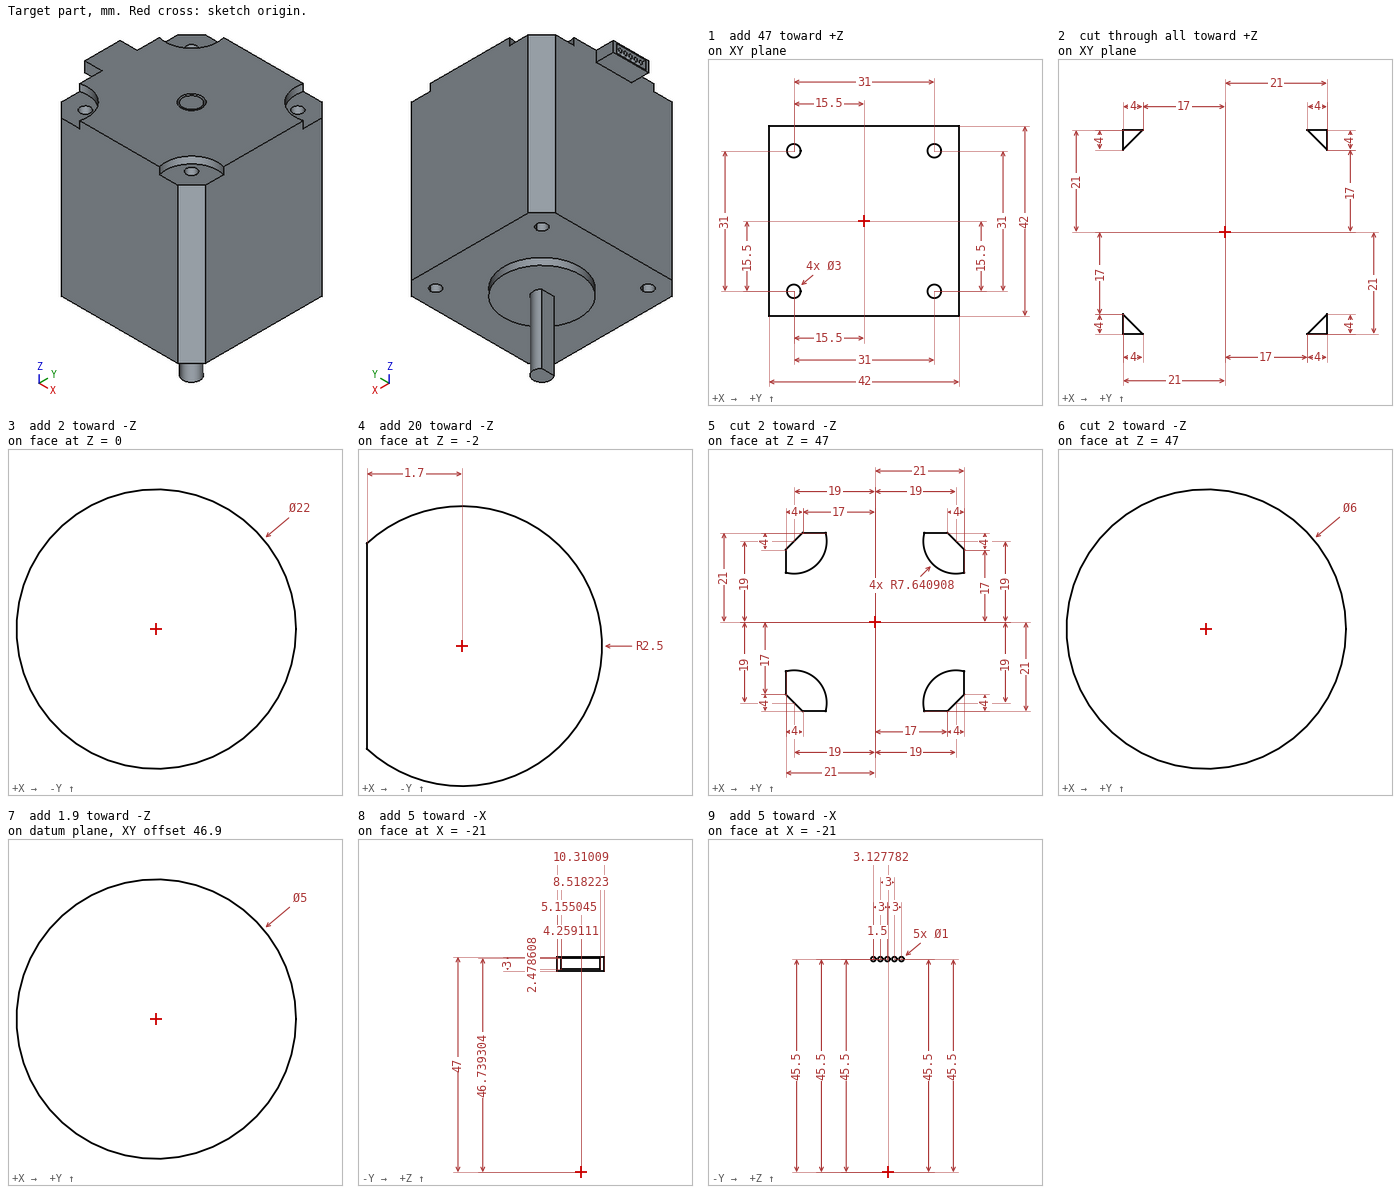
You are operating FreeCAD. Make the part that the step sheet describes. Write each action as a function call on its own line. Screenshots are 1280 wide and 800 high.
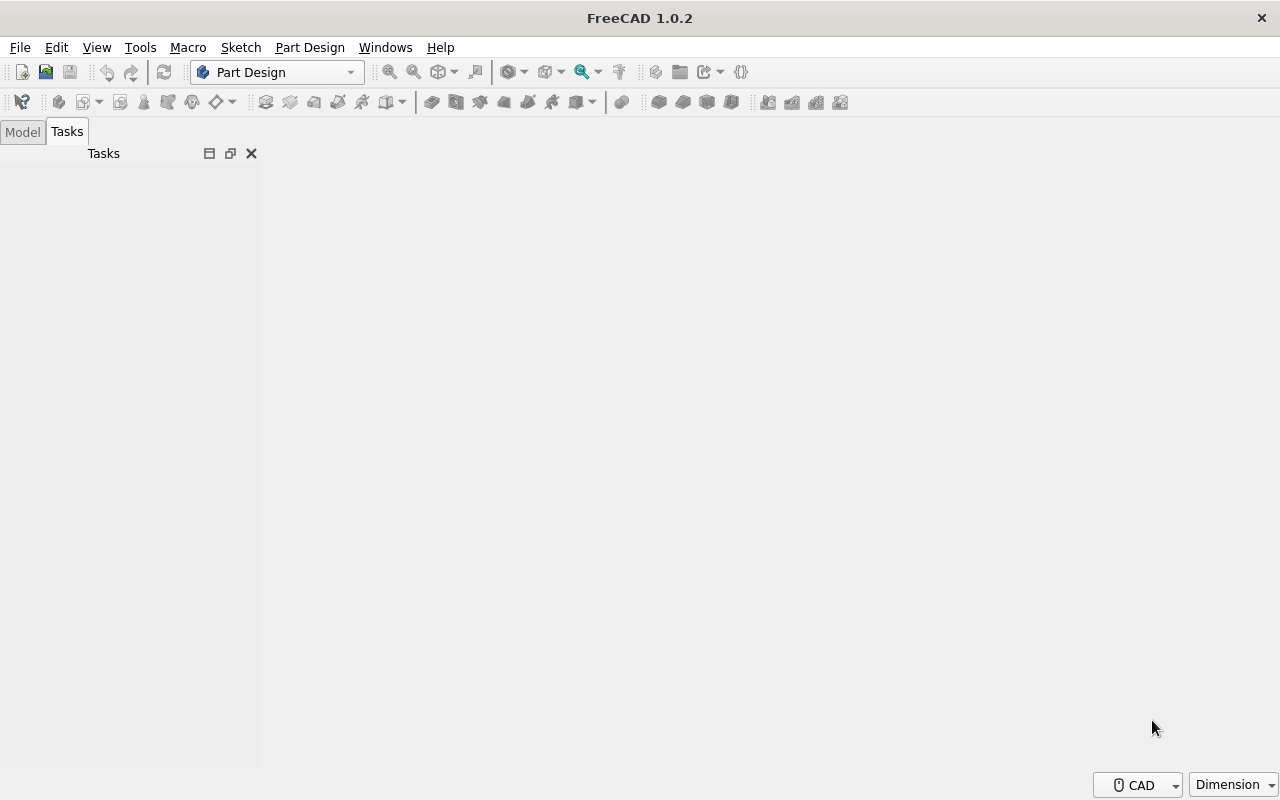
click(22, 72)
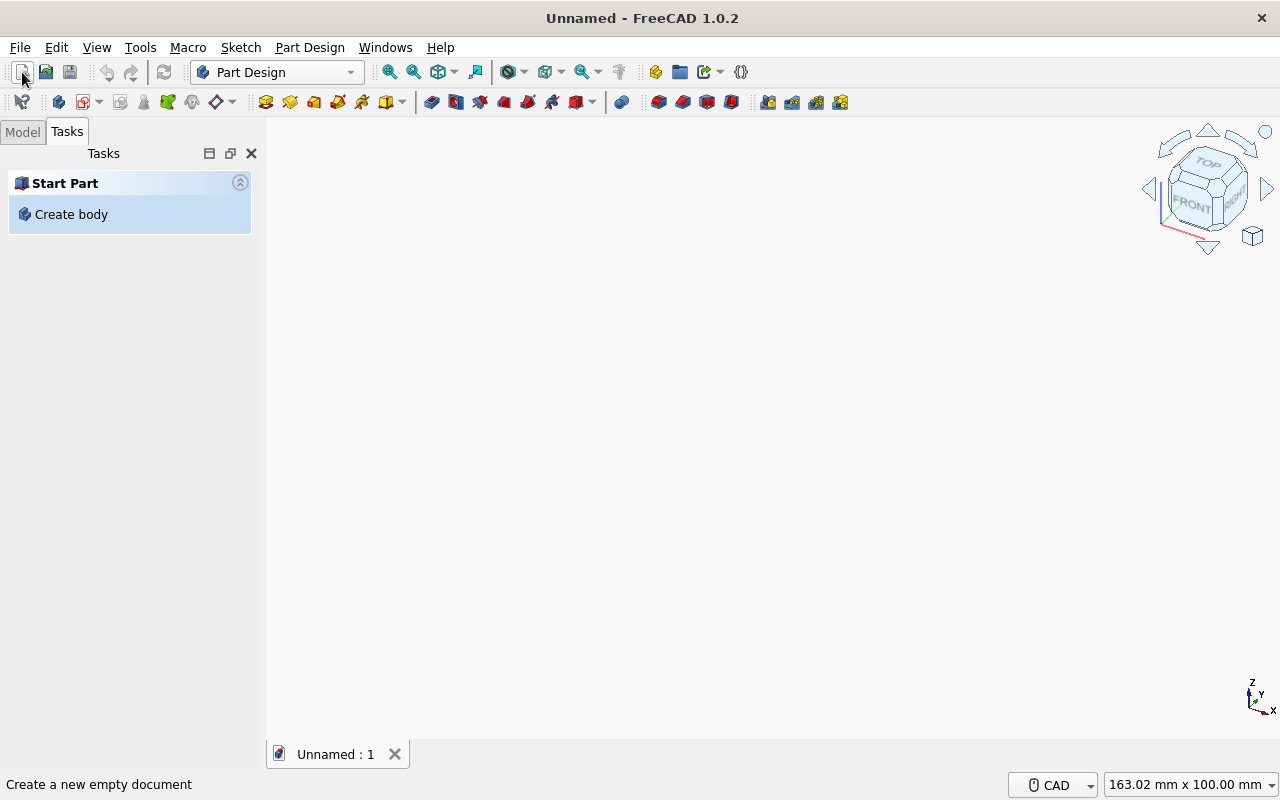
click(84, 102)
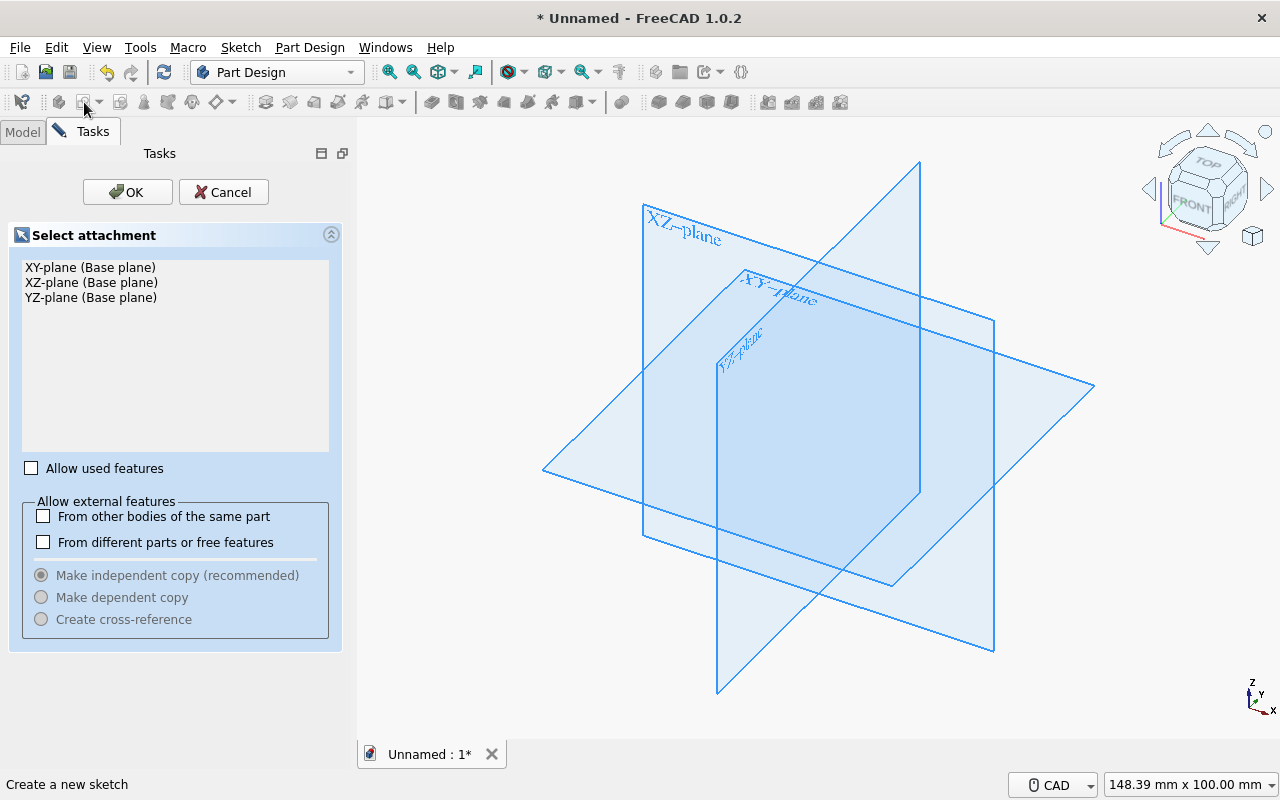
click(82, 268)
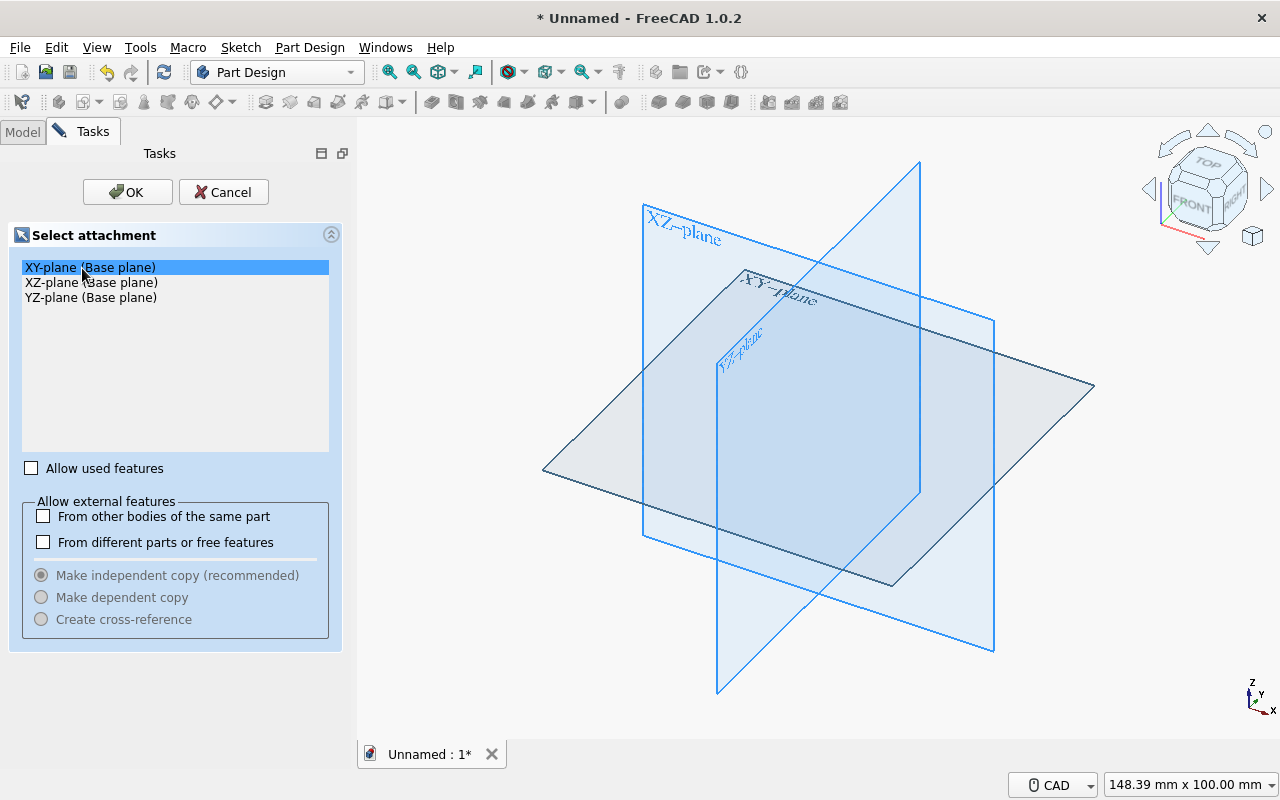
click(128, 192)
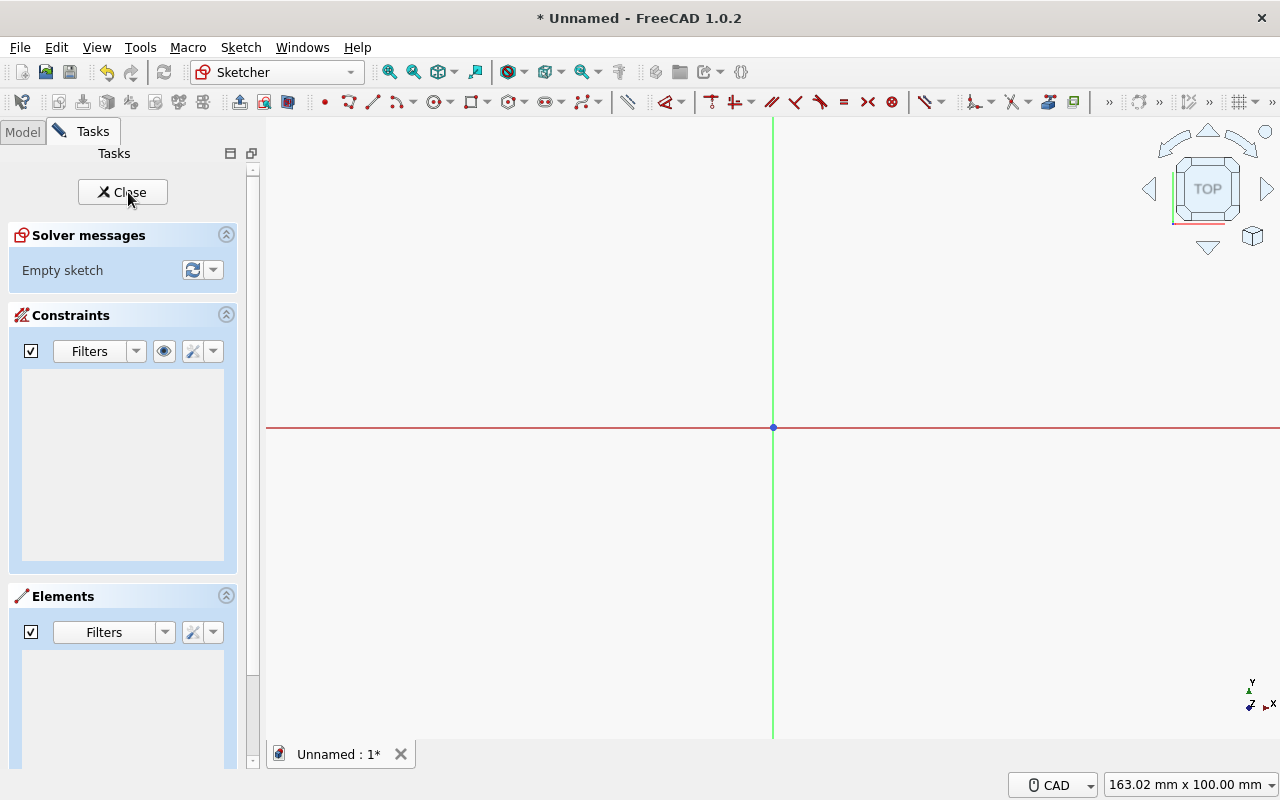
scroll(912, 428, up, 2)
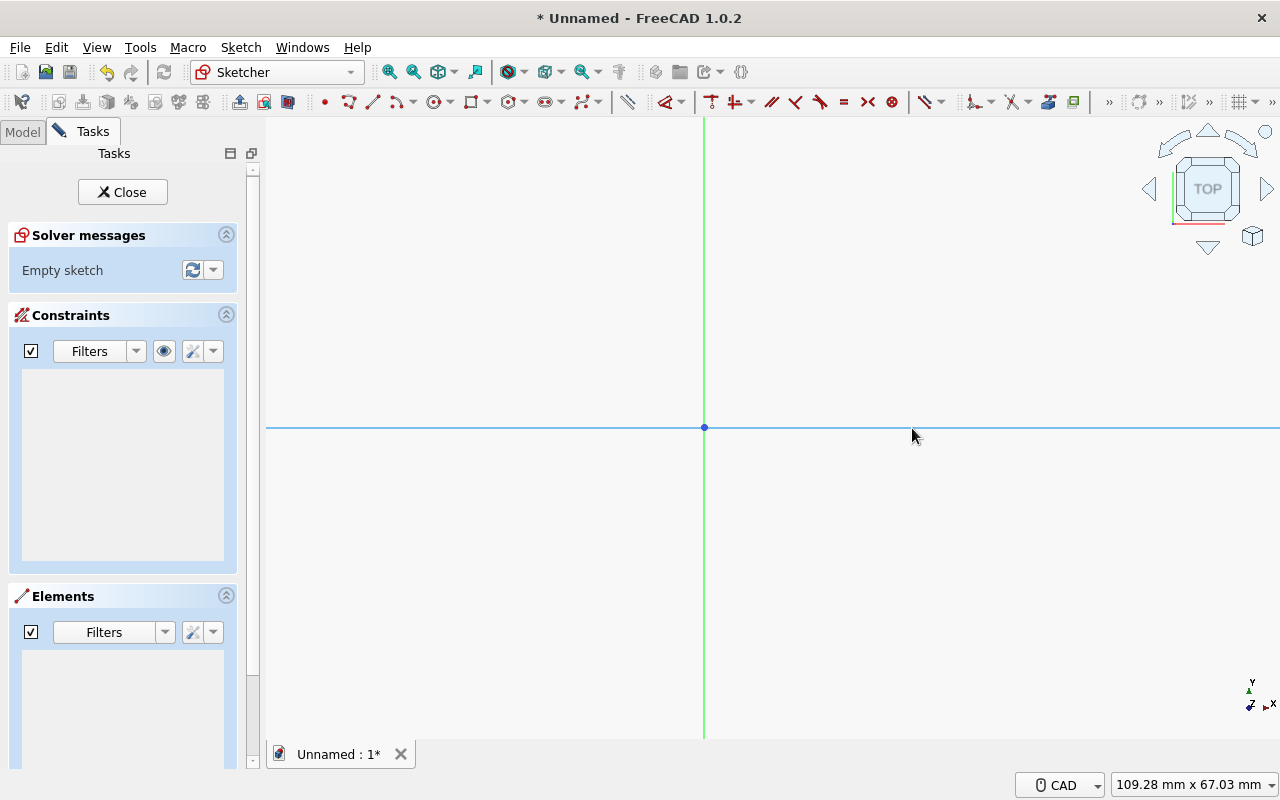
key(g)
key(v)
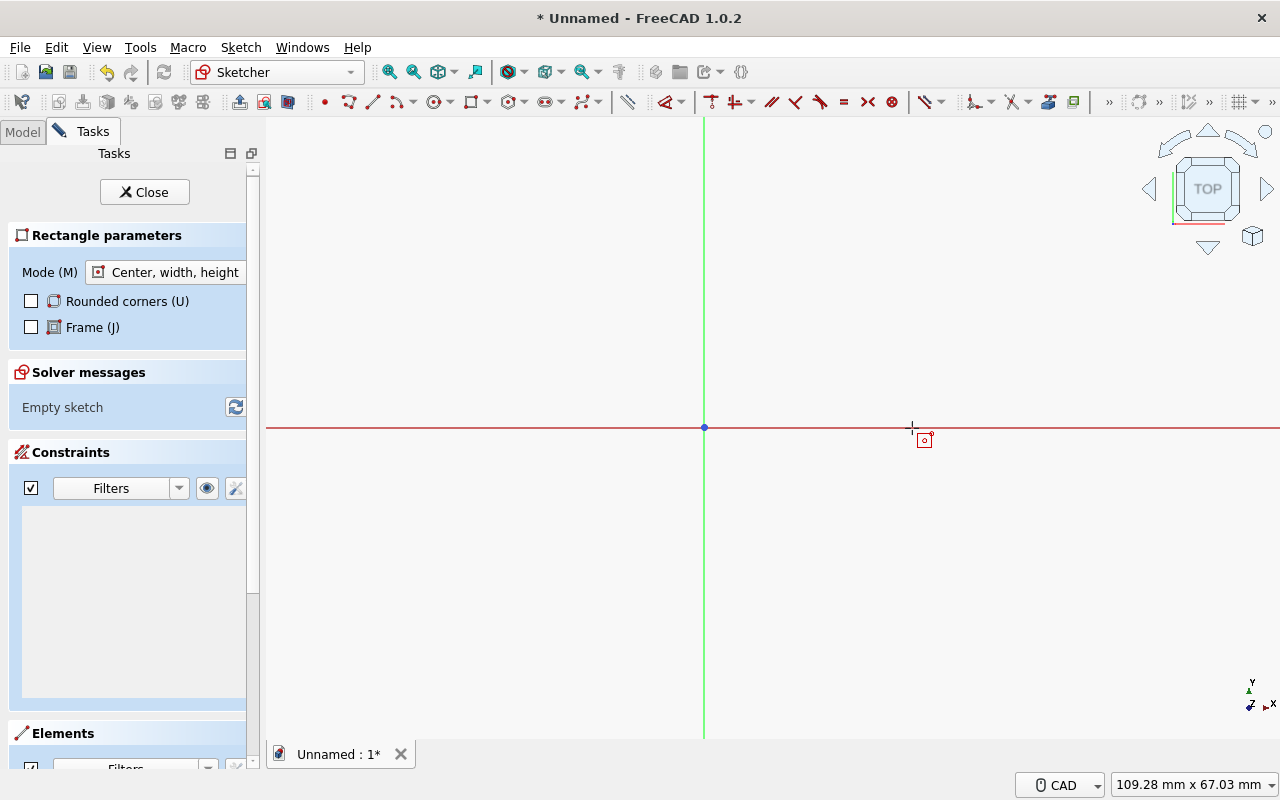
click(704, 428)
click(899, 233)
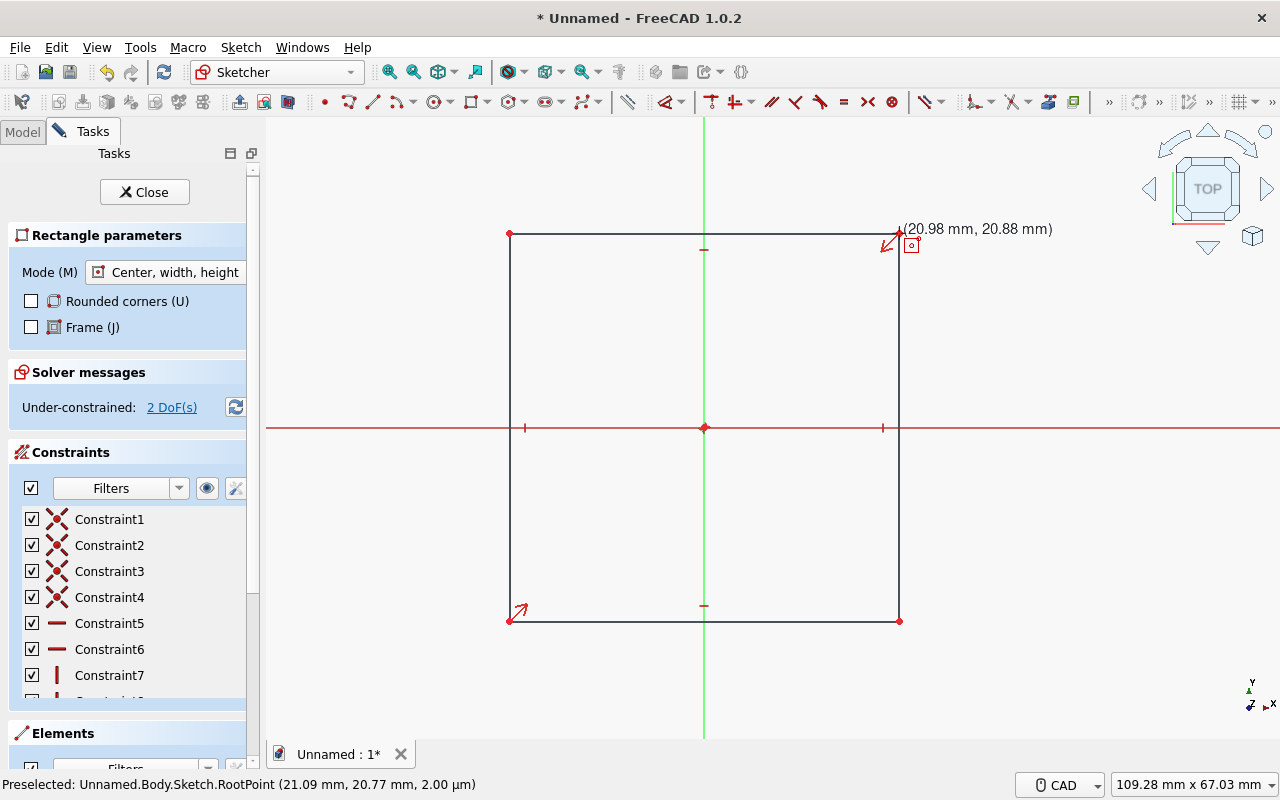
click(434, 102)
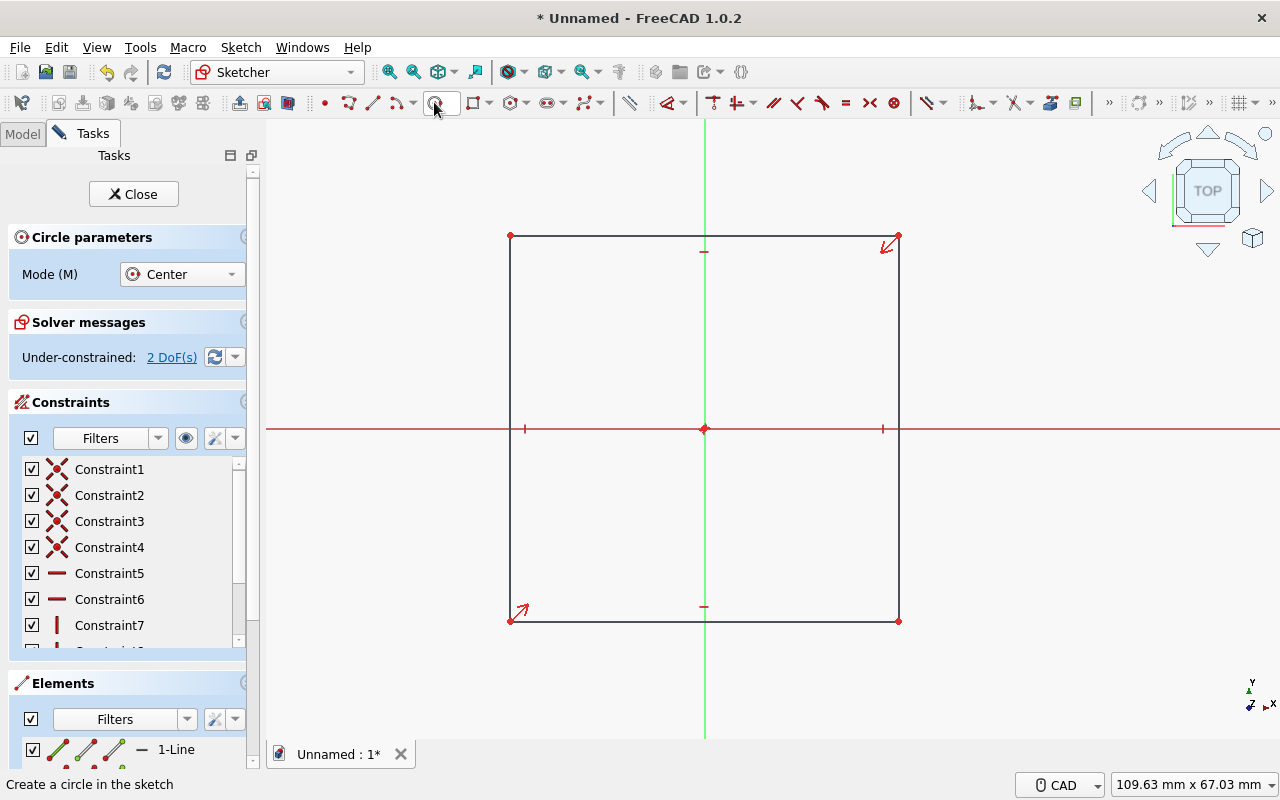
scroll(561, 572, up, 3)